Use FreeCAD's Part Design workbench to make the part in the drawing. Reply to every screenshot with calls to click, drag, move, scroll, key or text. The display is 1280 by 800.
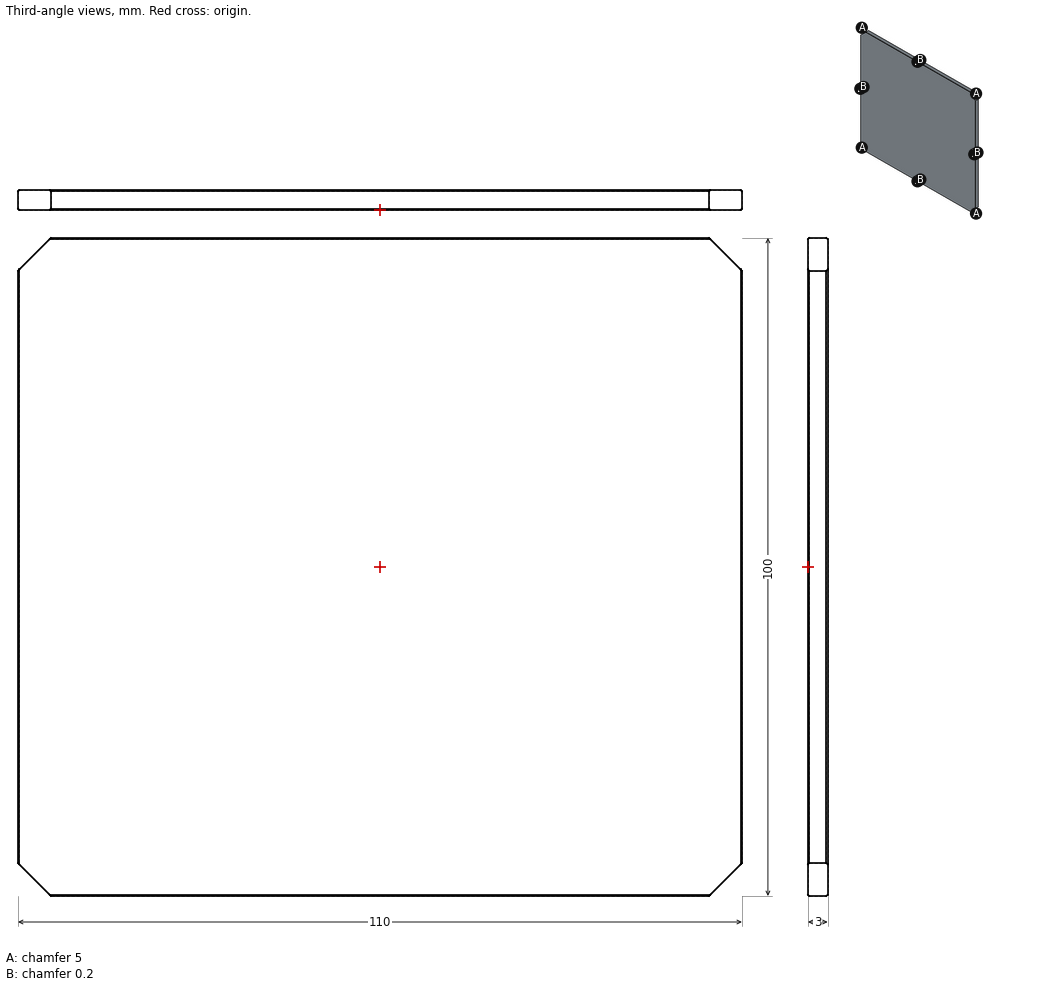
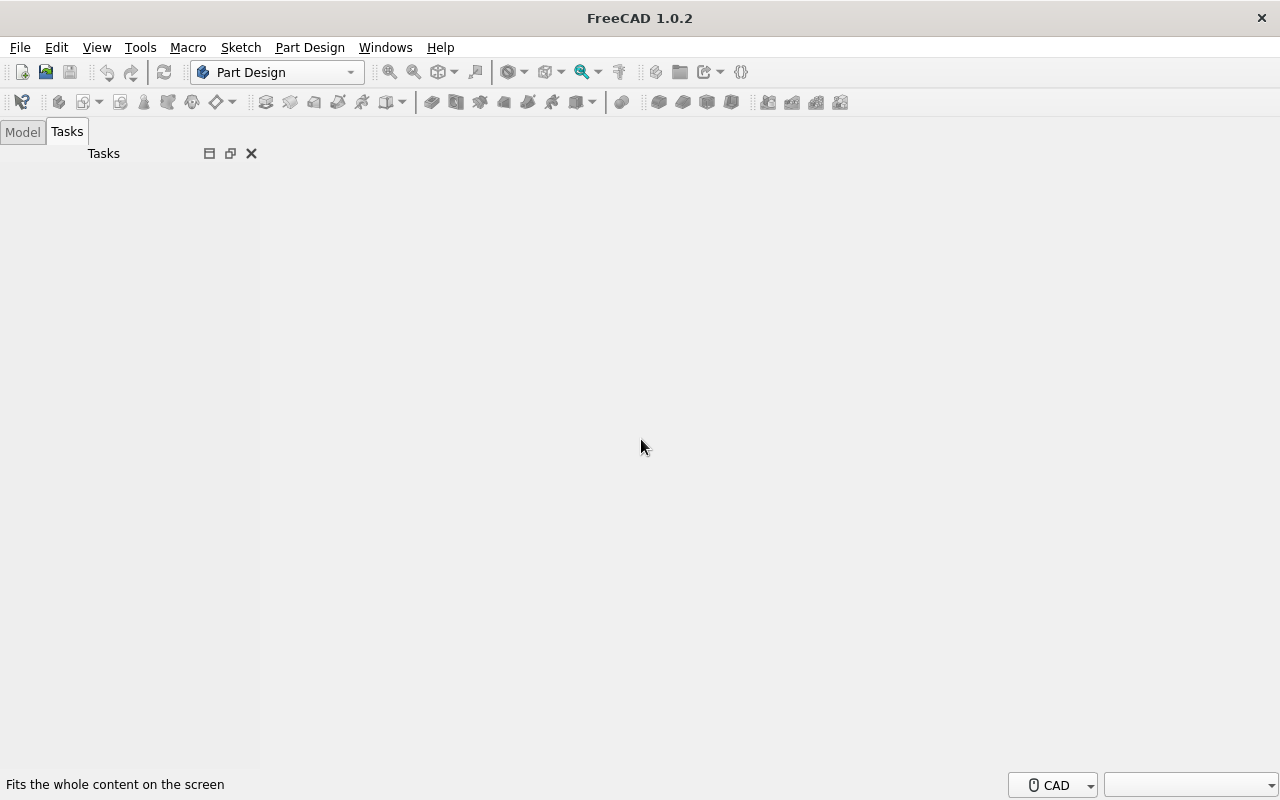
click(22, 72)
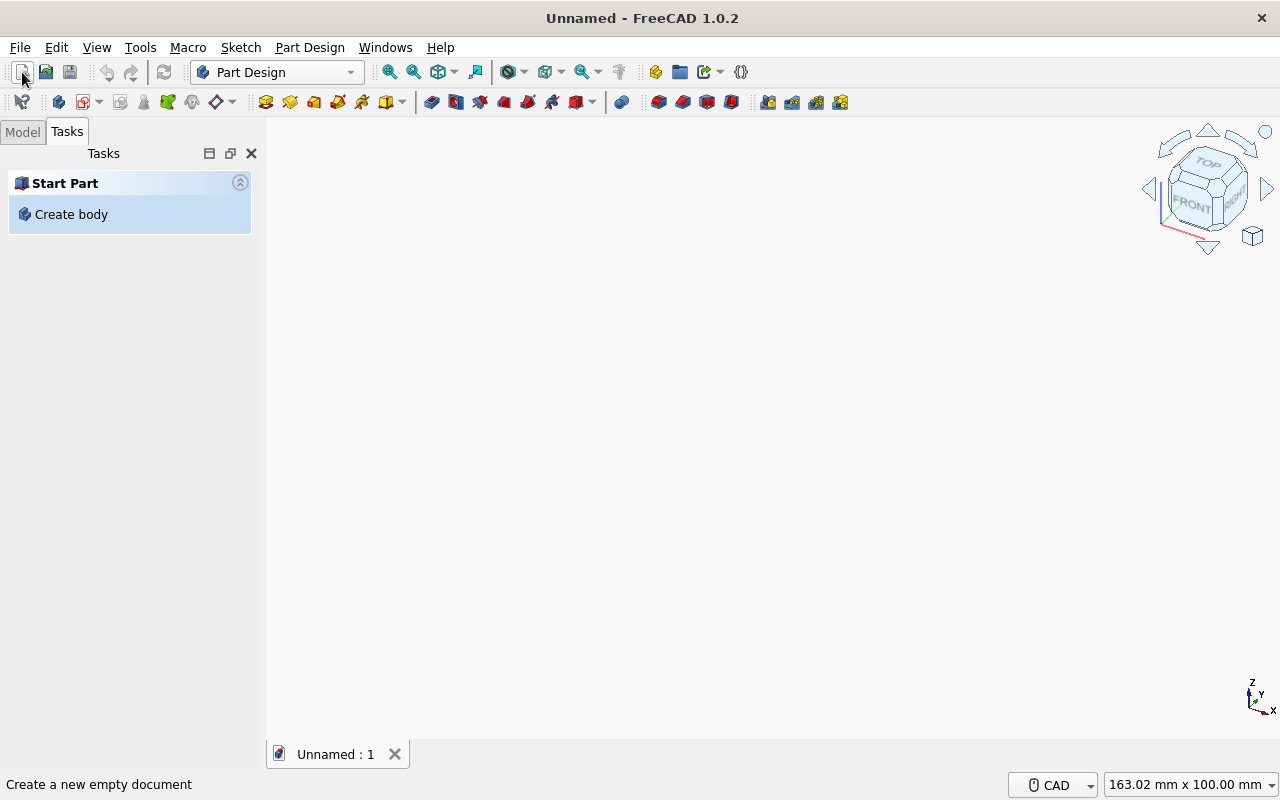
click(84, 102)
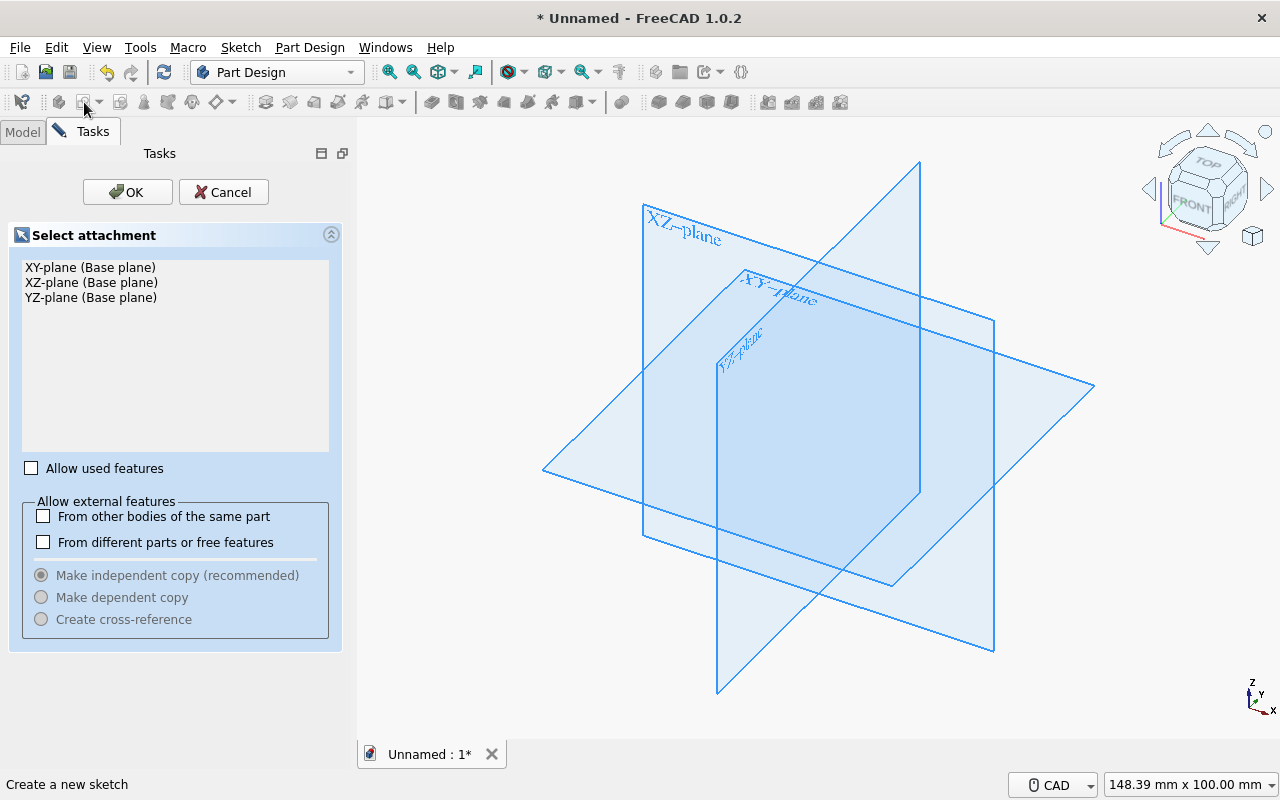
click(82, 282)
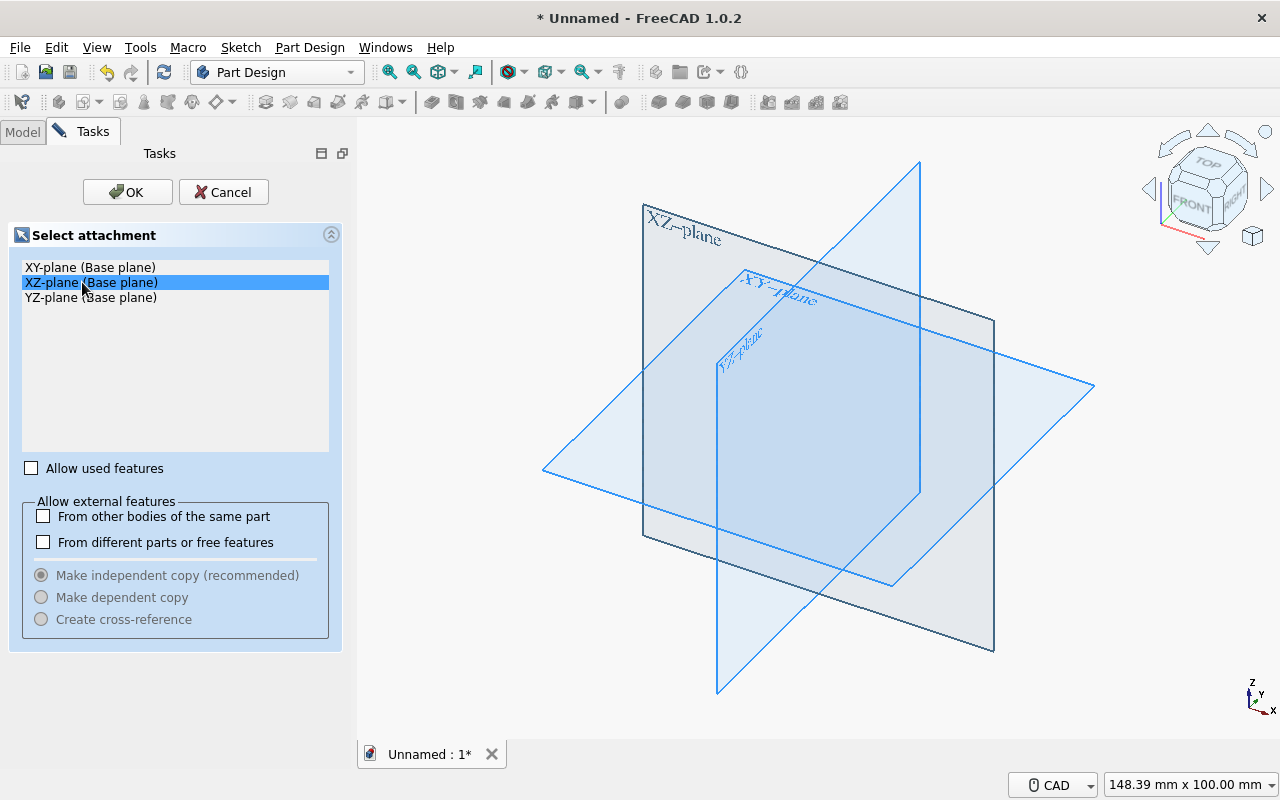
click(128, 192)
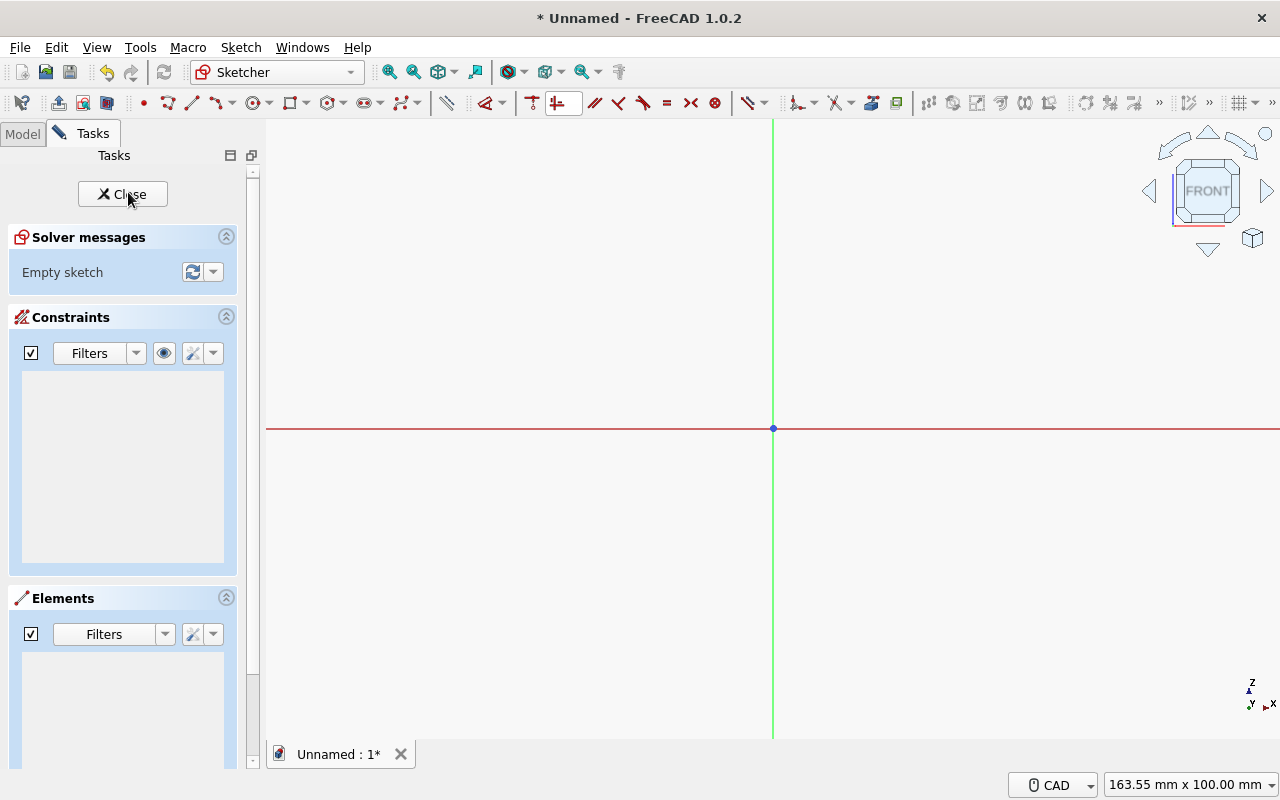
scroll(565, 429, down, 2)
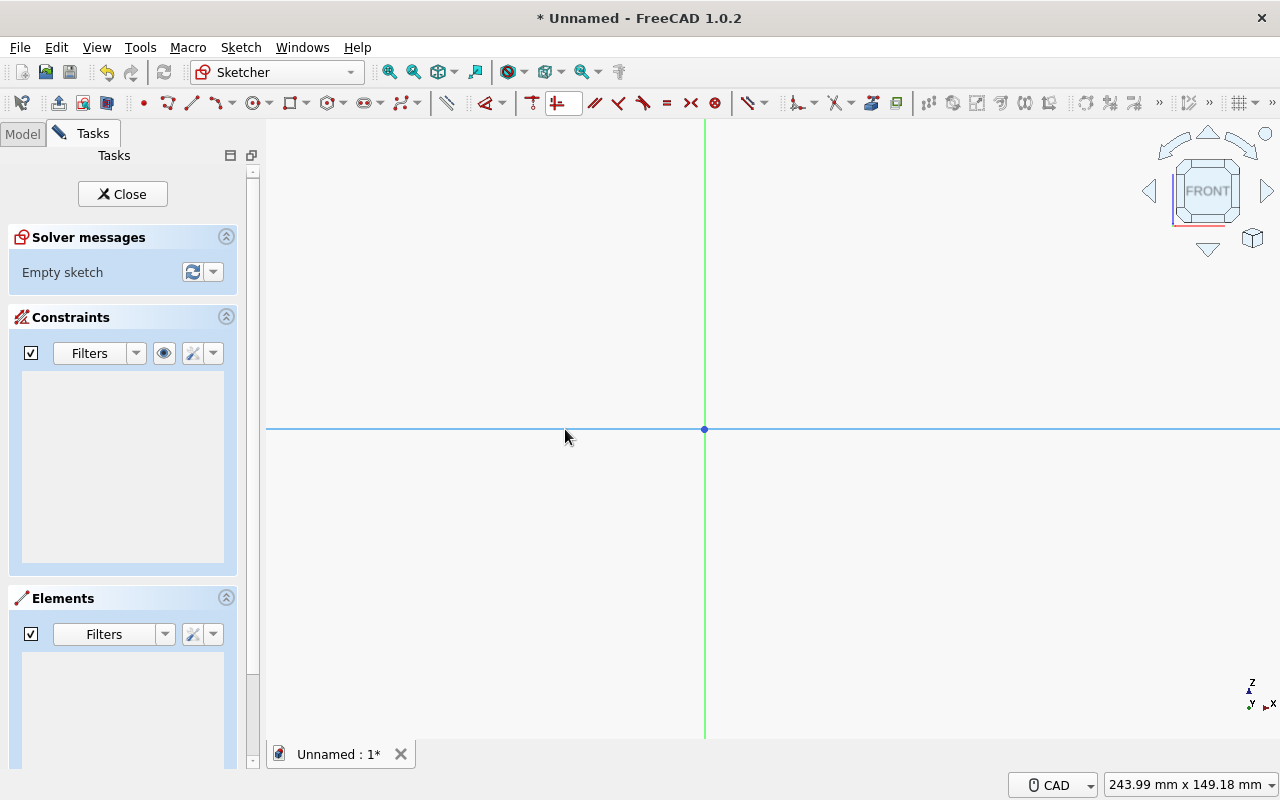
key(g)
key(v)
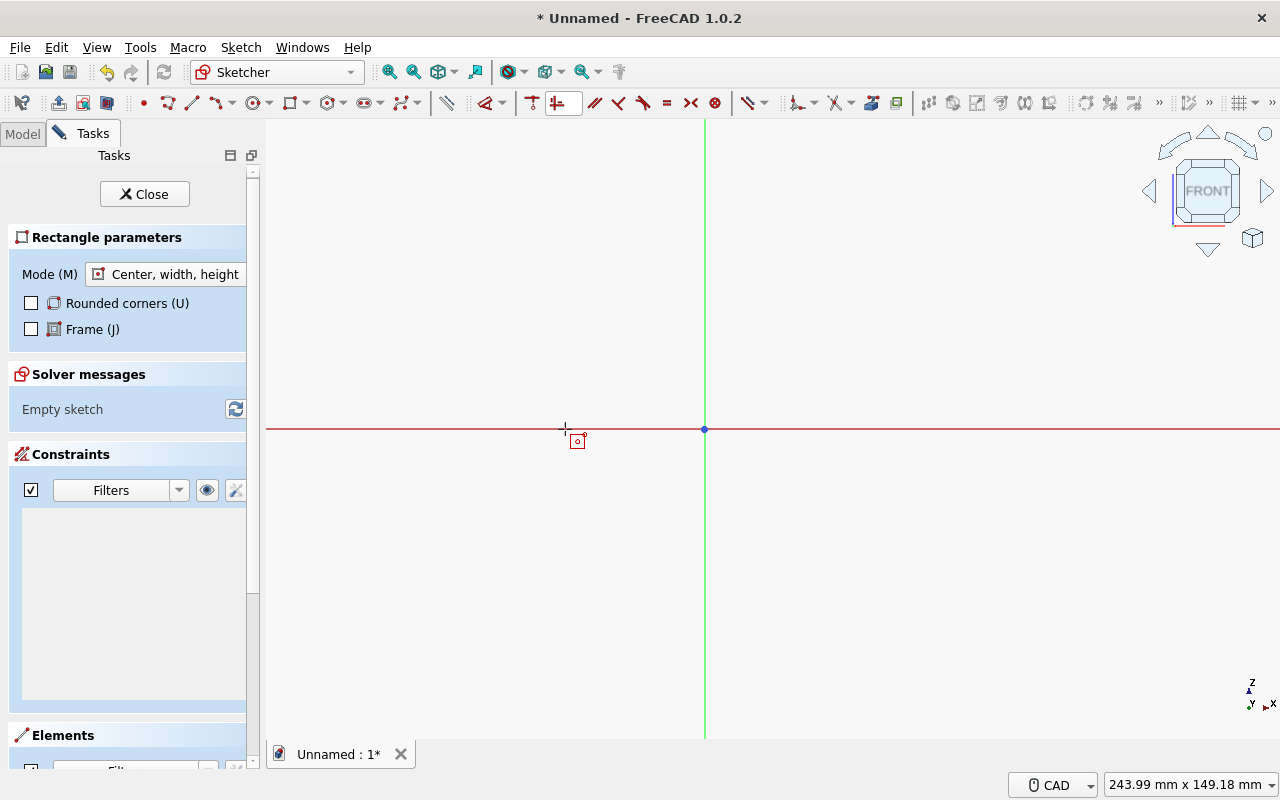
click(705, 429)
click(933, 221)
key(Escape)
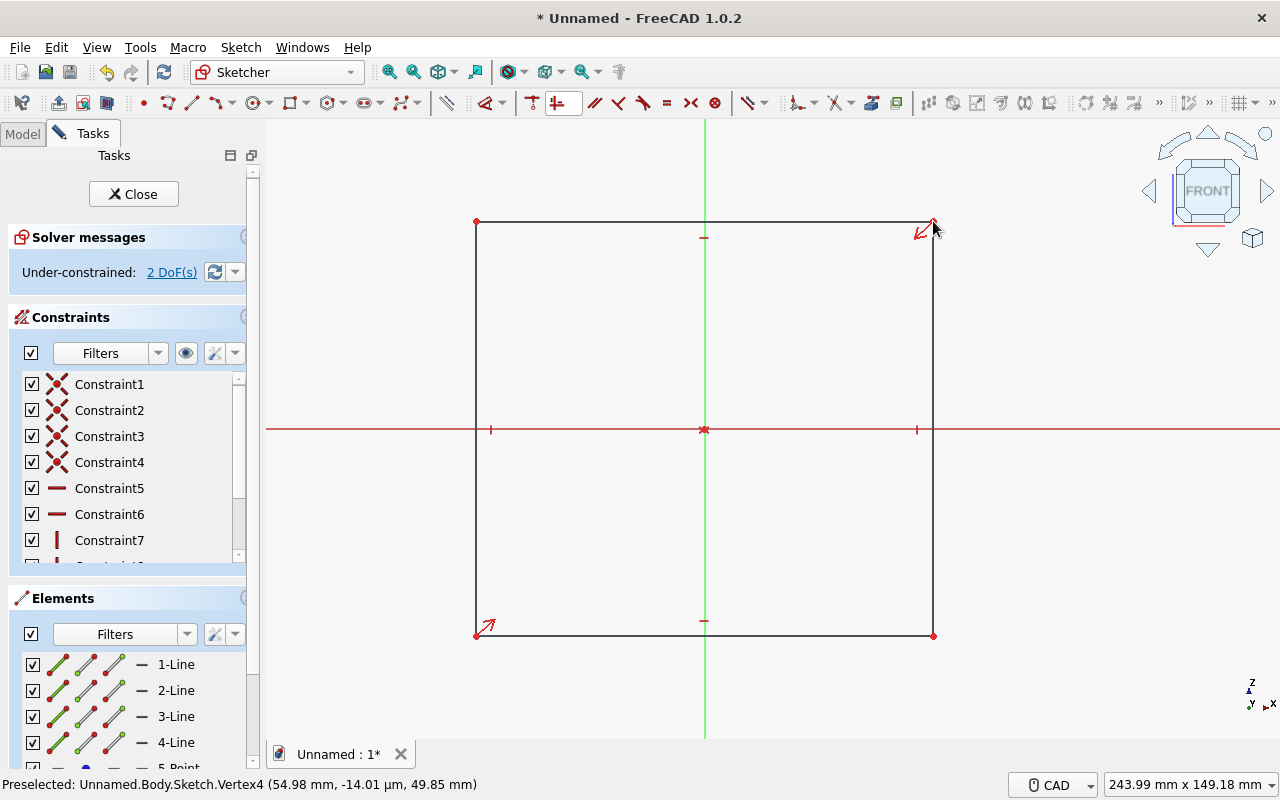
click(613, 636)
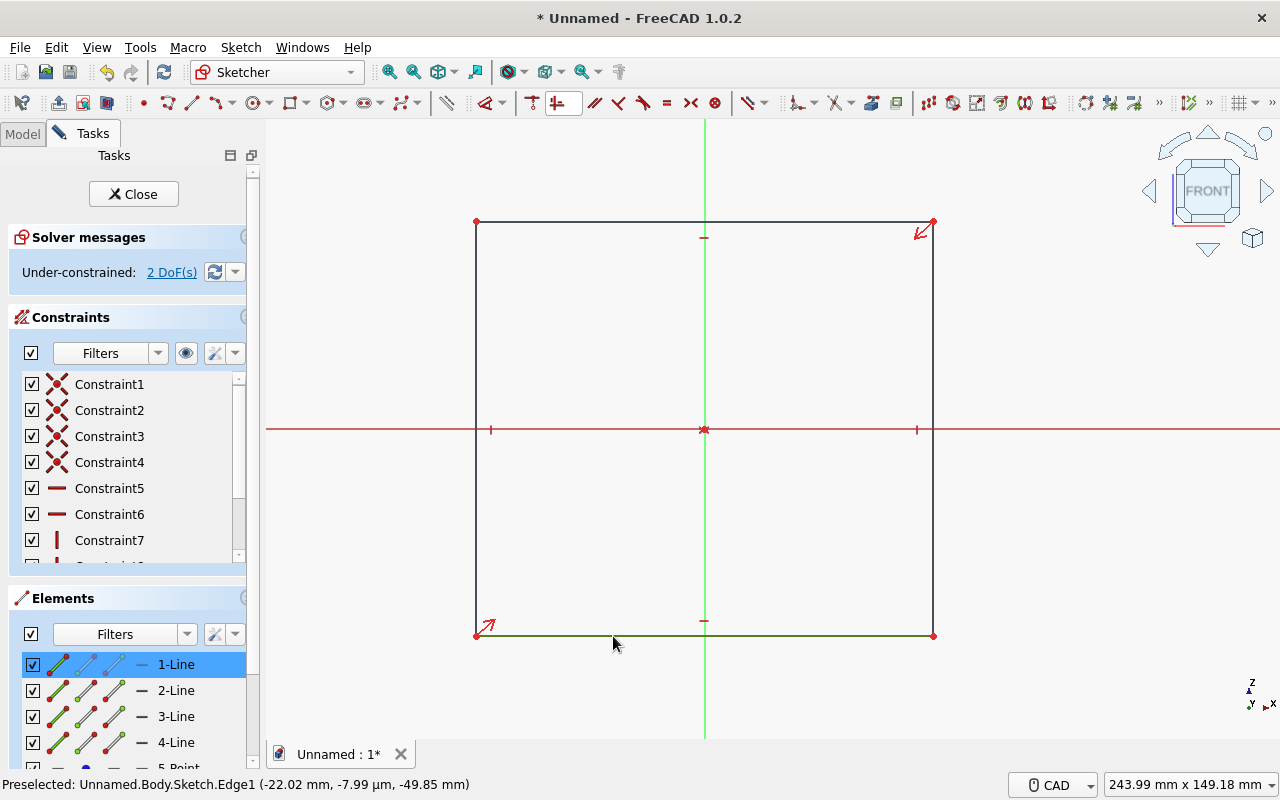
key(l)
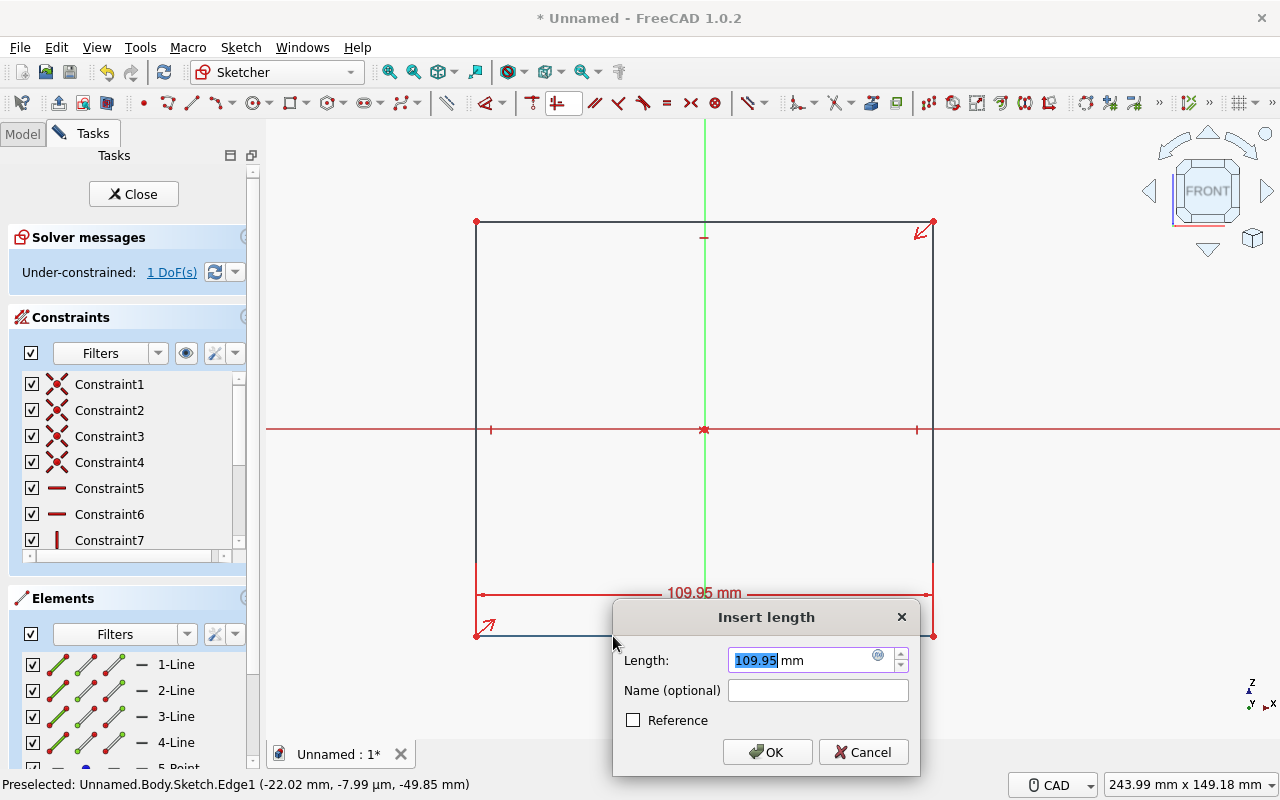
text(110)
key(Return)